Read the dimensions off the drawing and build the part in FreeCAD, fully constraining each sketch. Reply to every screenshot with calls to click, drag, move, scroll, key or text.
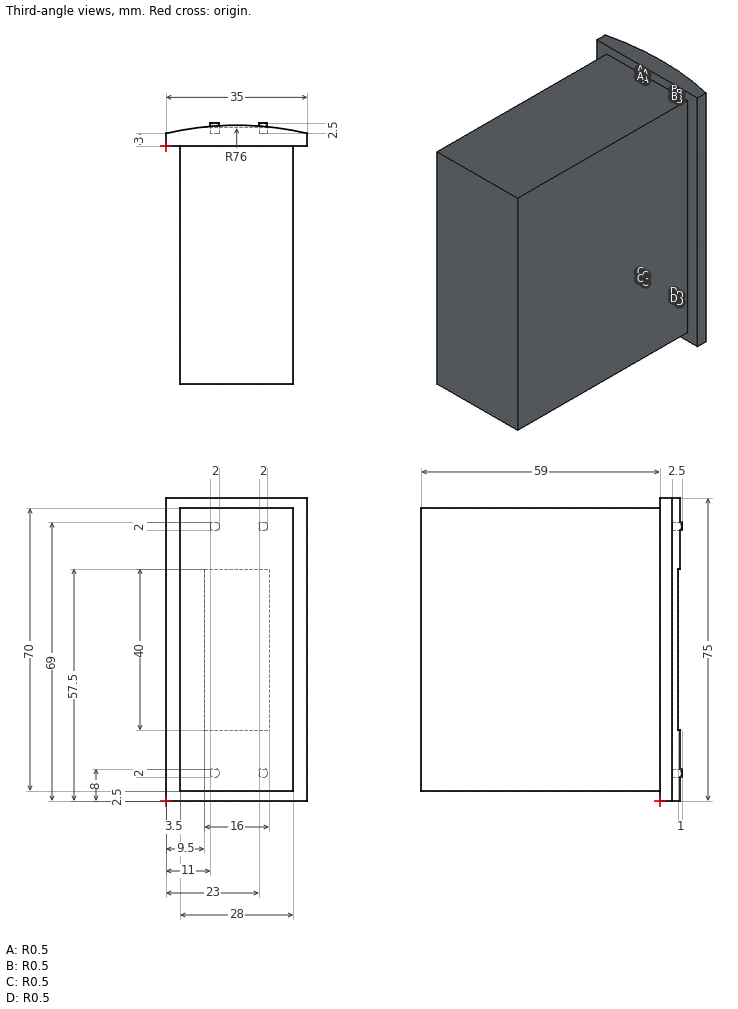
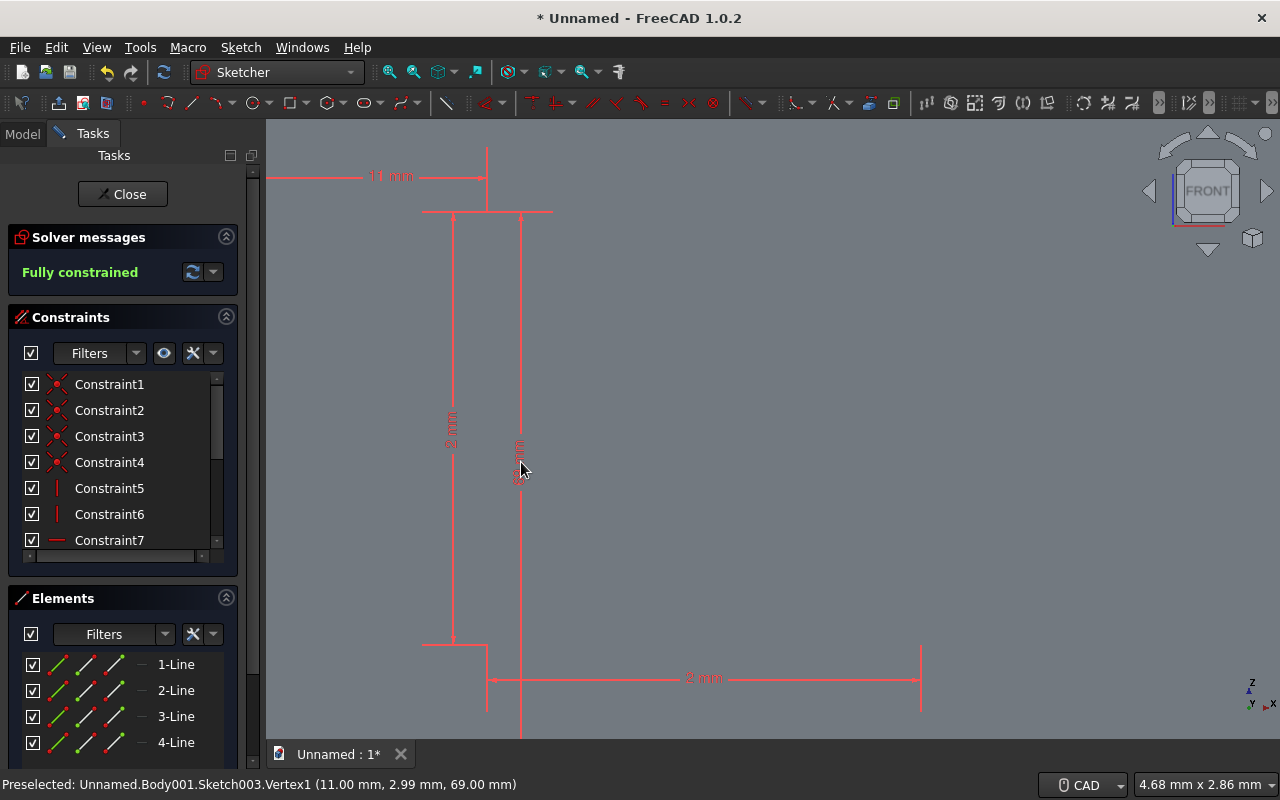
click(123, 194)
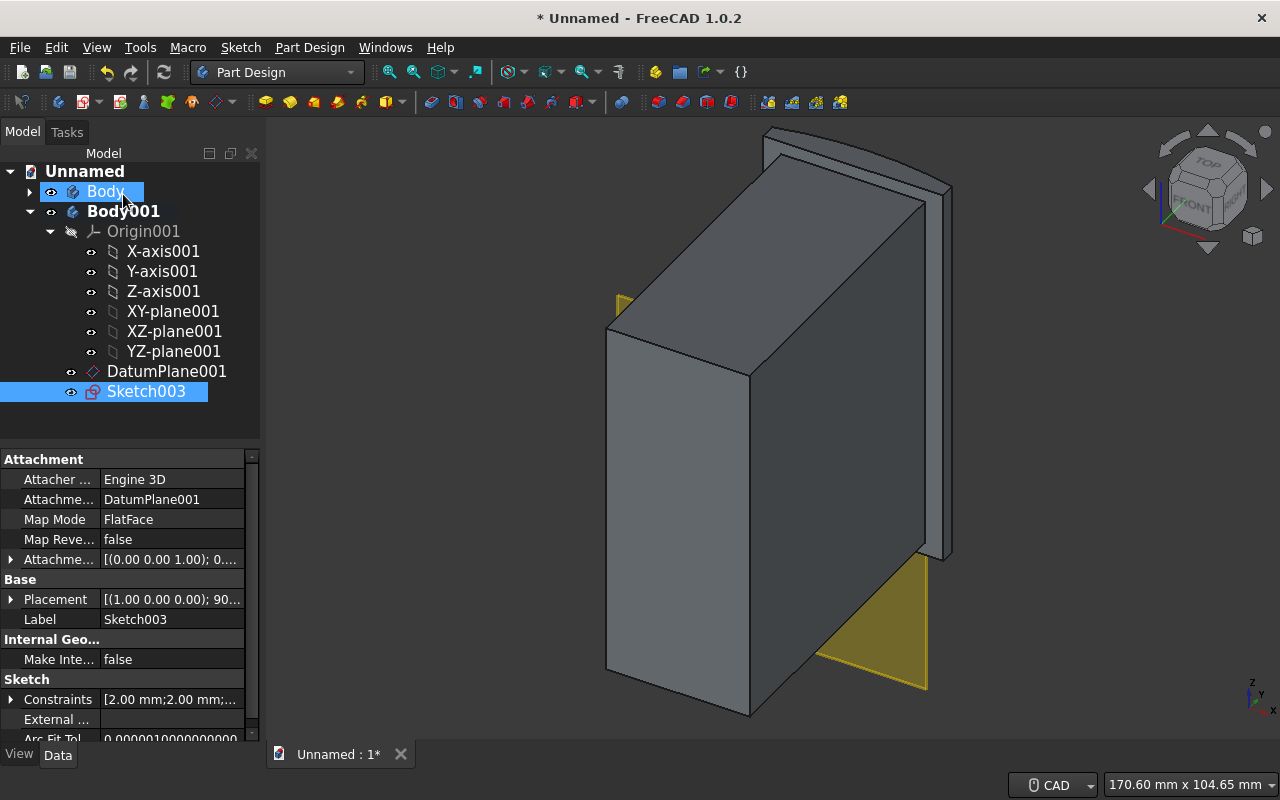
click(266, 102)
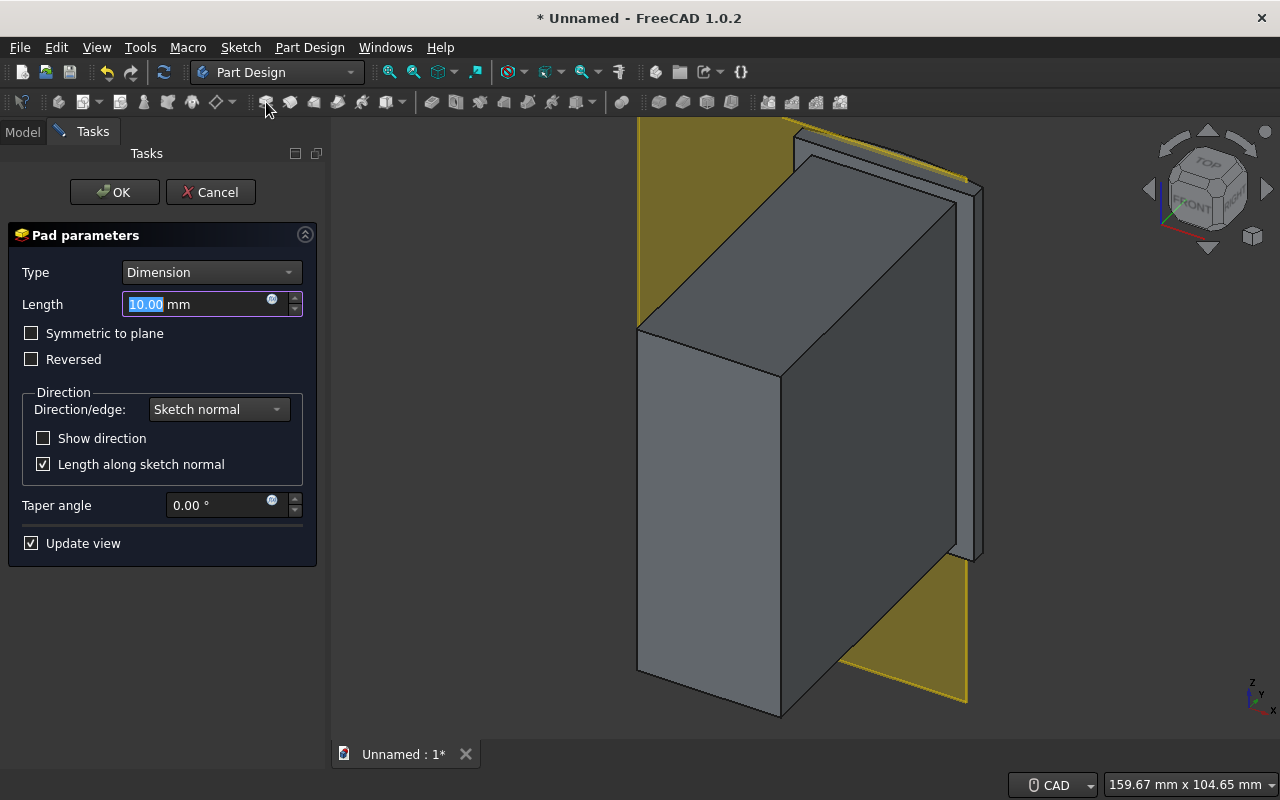
text(2.5)
key(Tab)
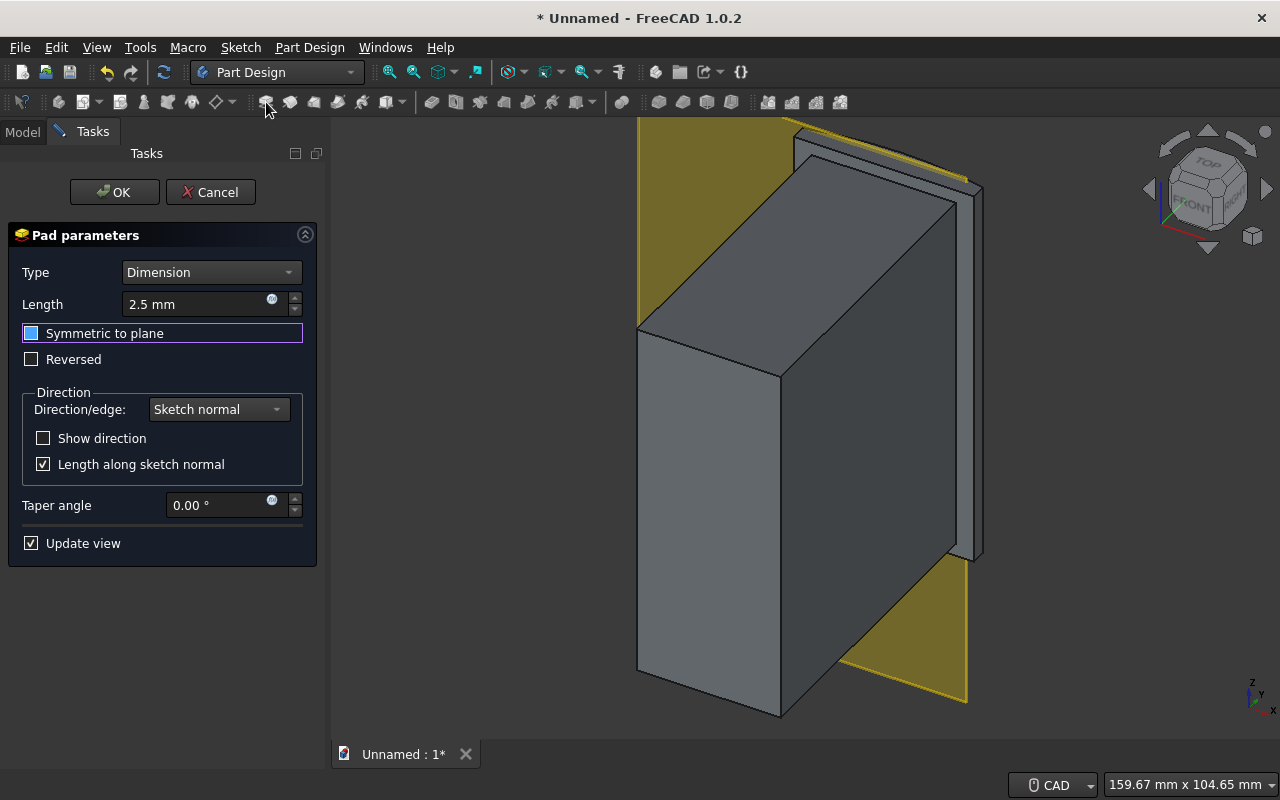
click(30, 359)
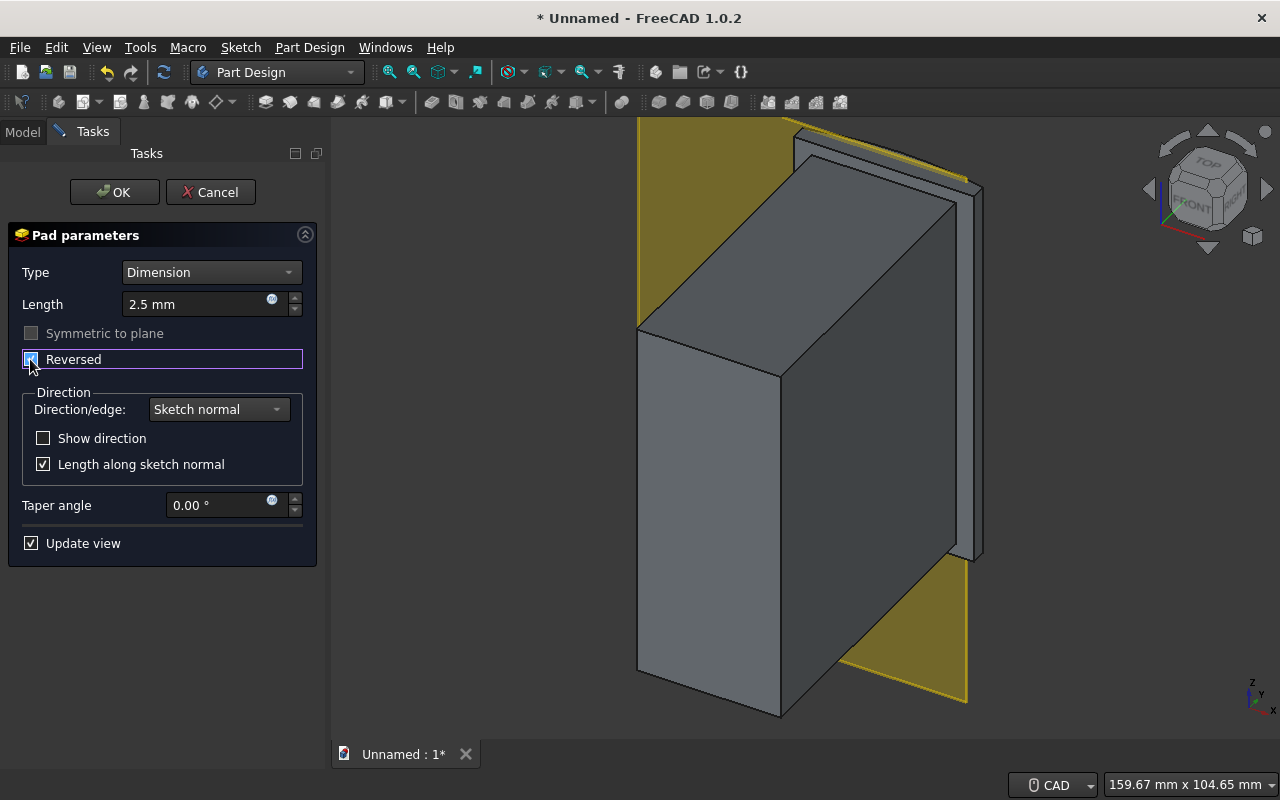
click(115, 192)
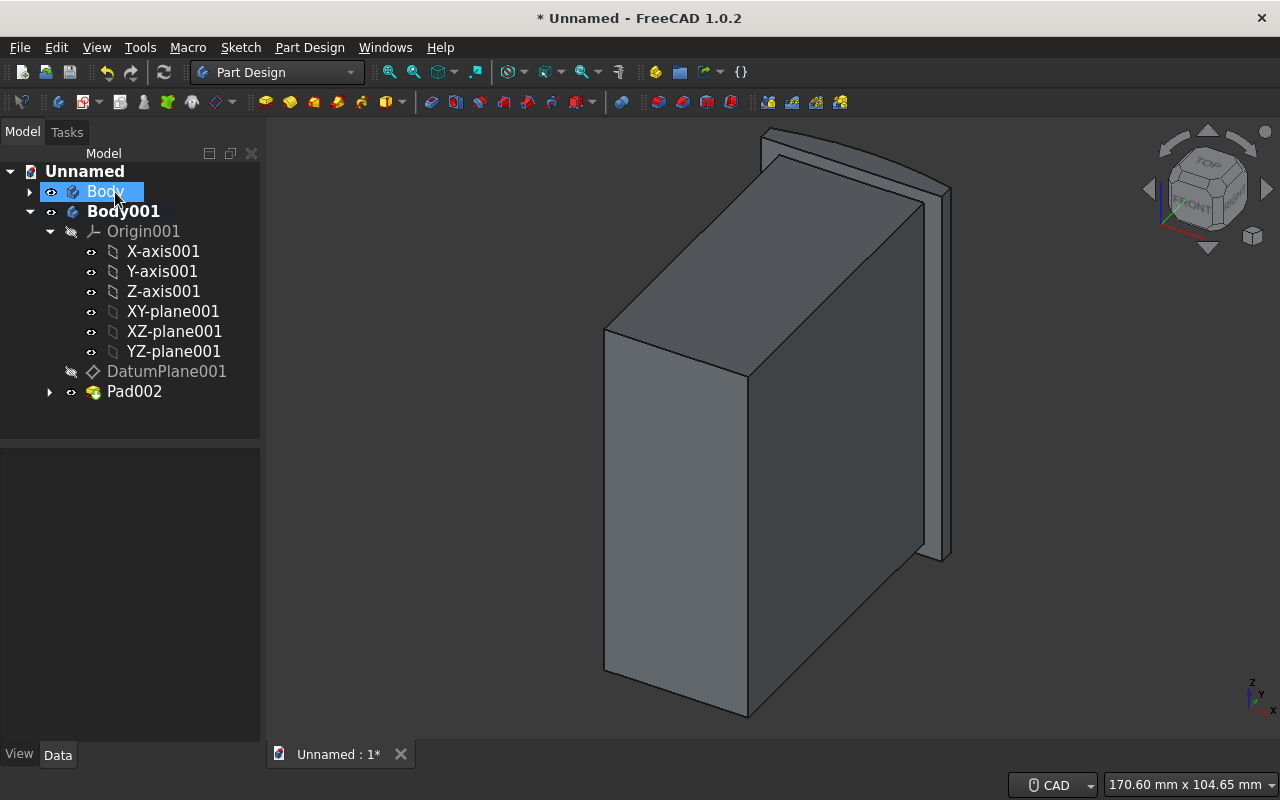
key(v)
key(f)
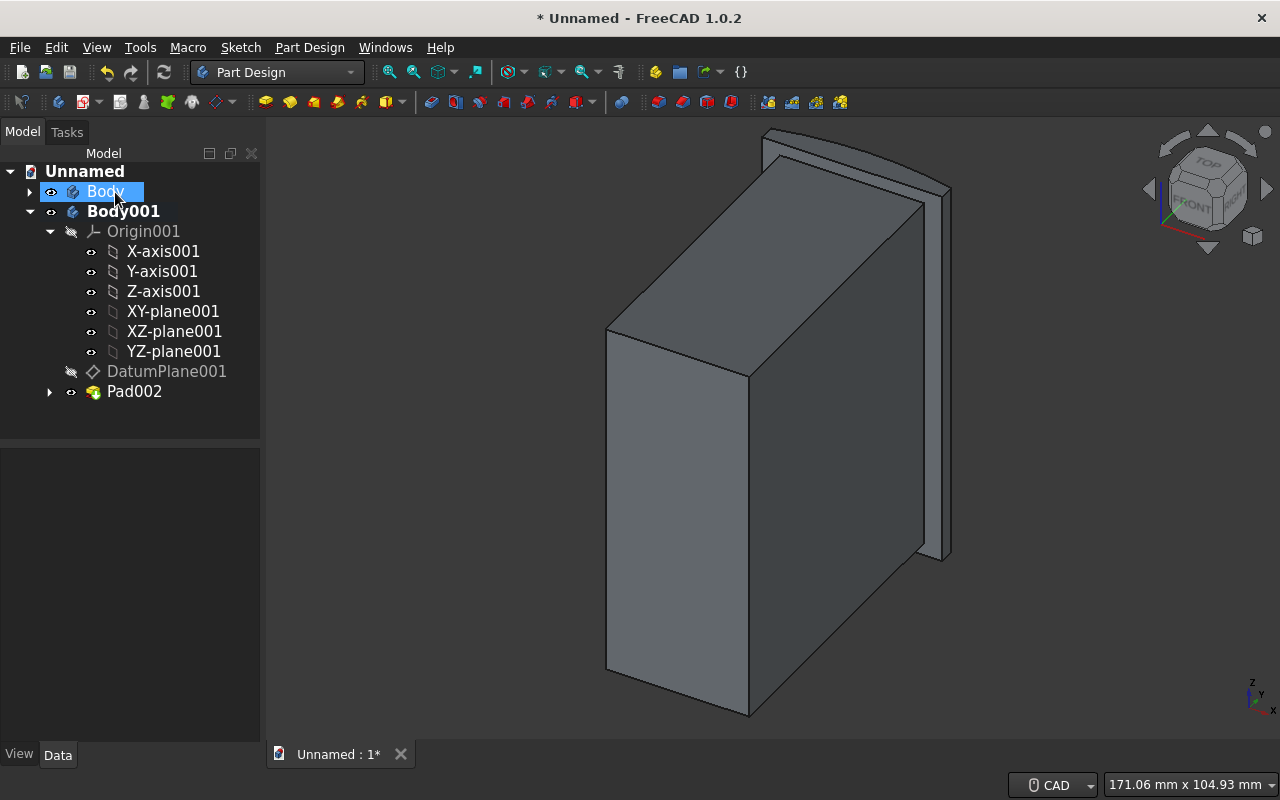
scroll(832, 172, up, 5)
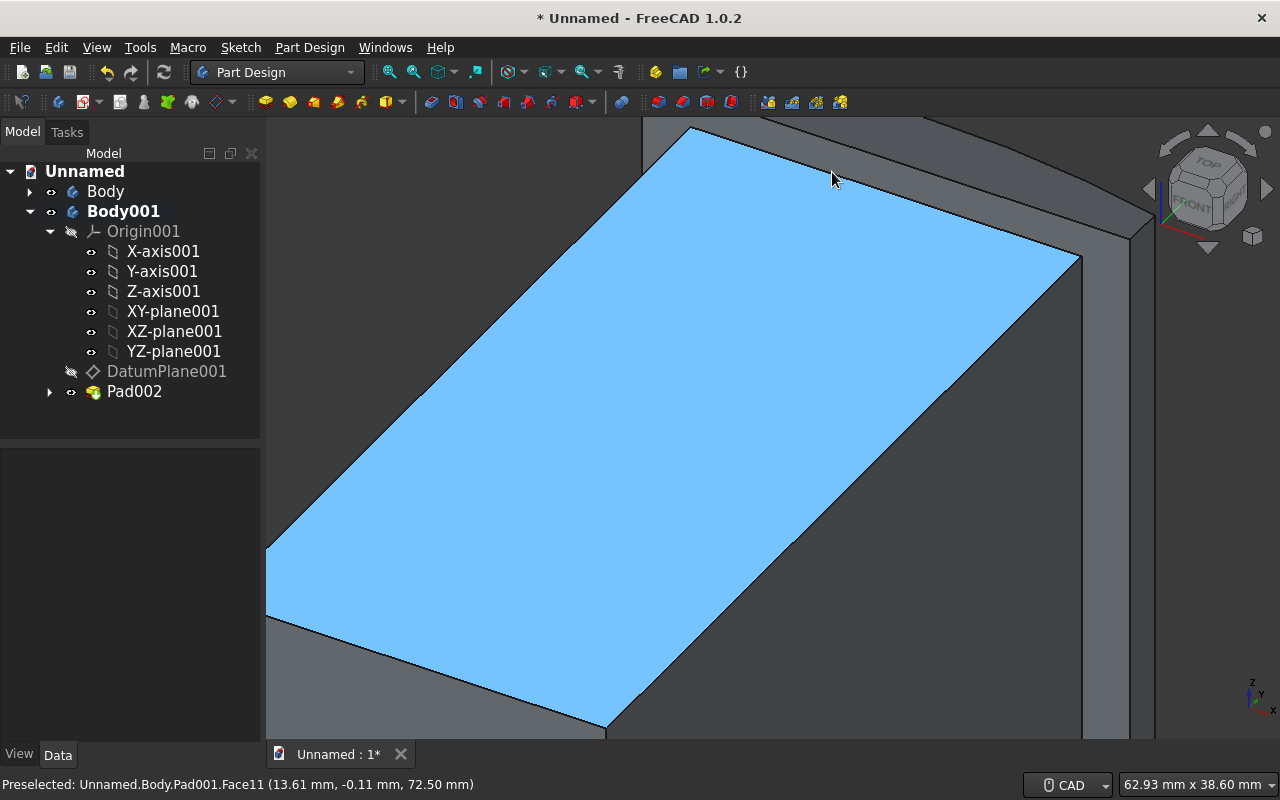
click(390, 72)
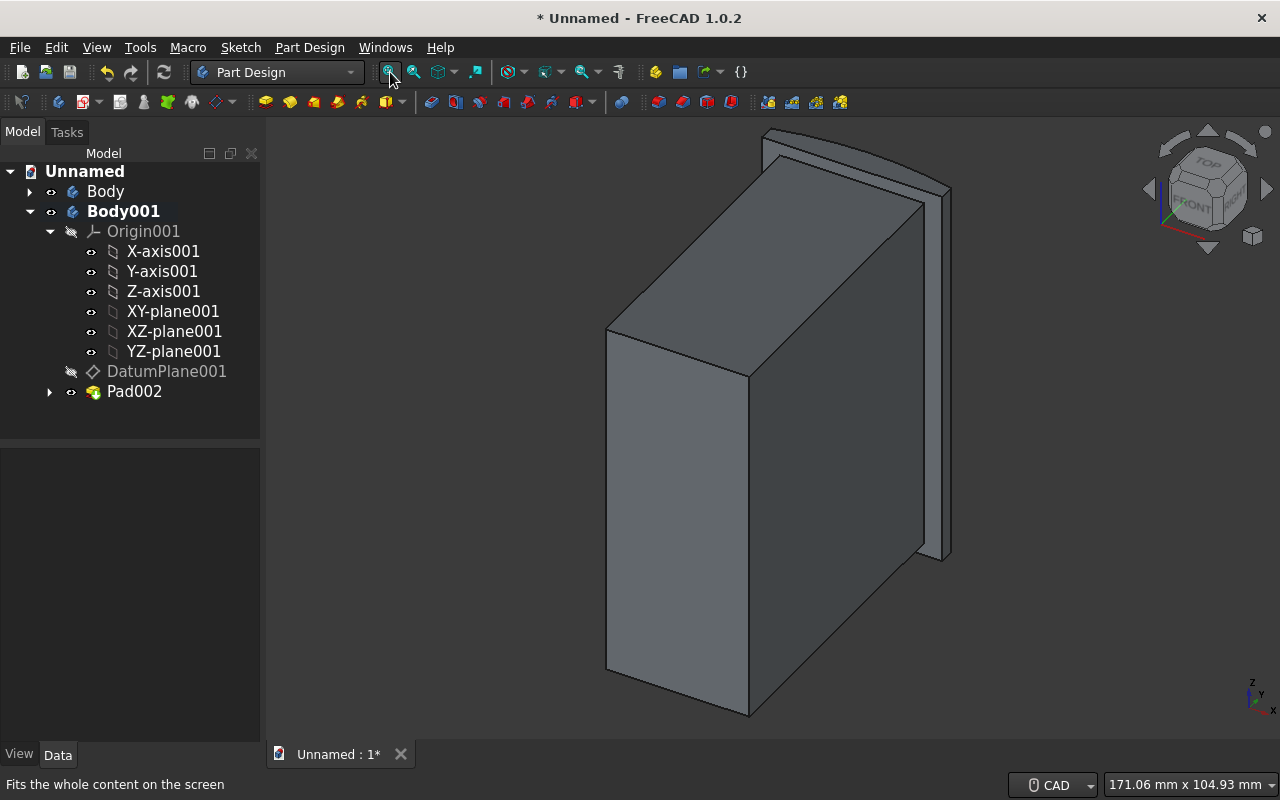
key(0)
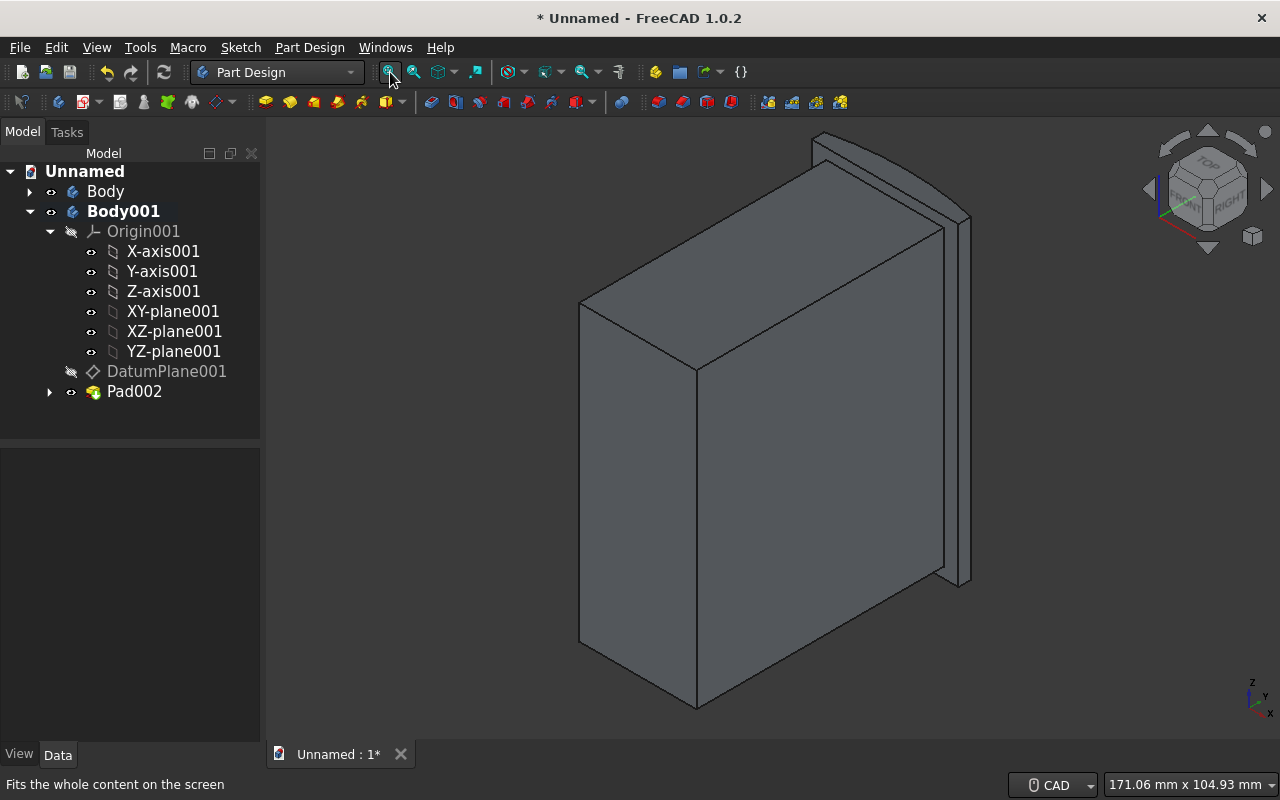
key(v)
key(f)